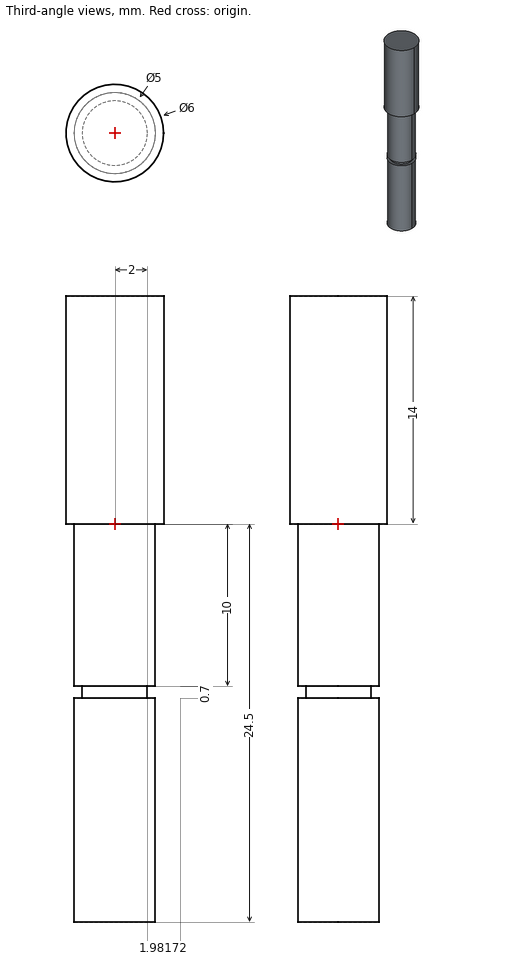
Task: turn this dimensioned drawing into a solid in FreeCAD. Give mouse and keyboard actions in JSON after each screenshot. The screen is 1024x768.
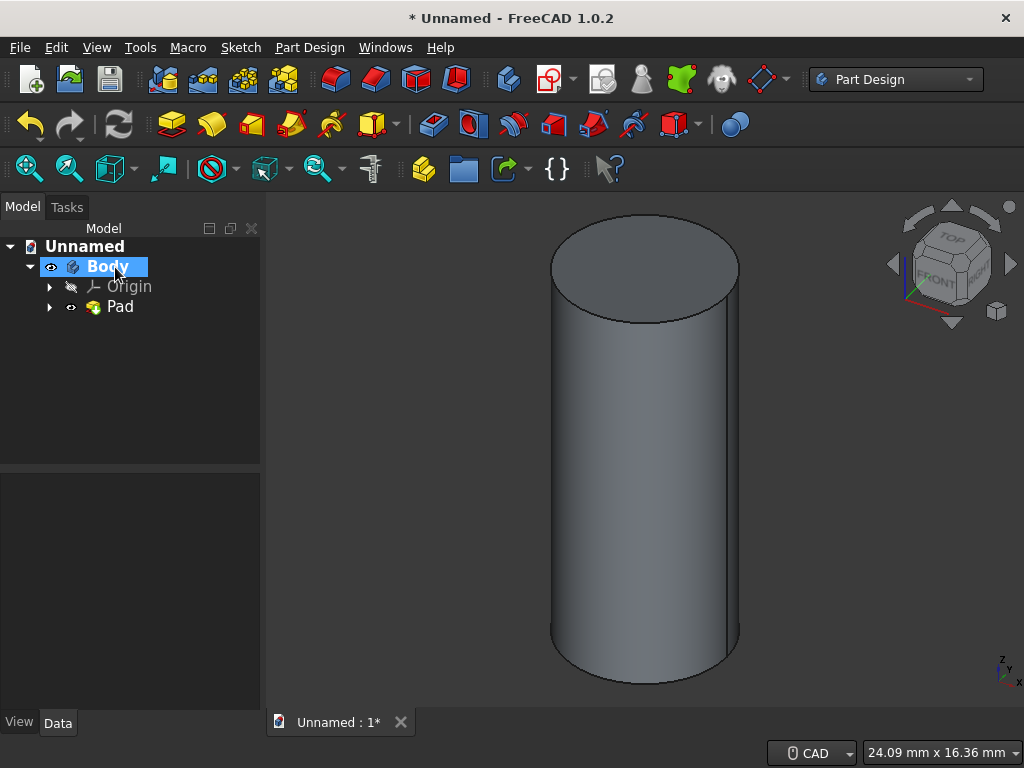
{"action": "left_click", "coordinate": [550, 80]}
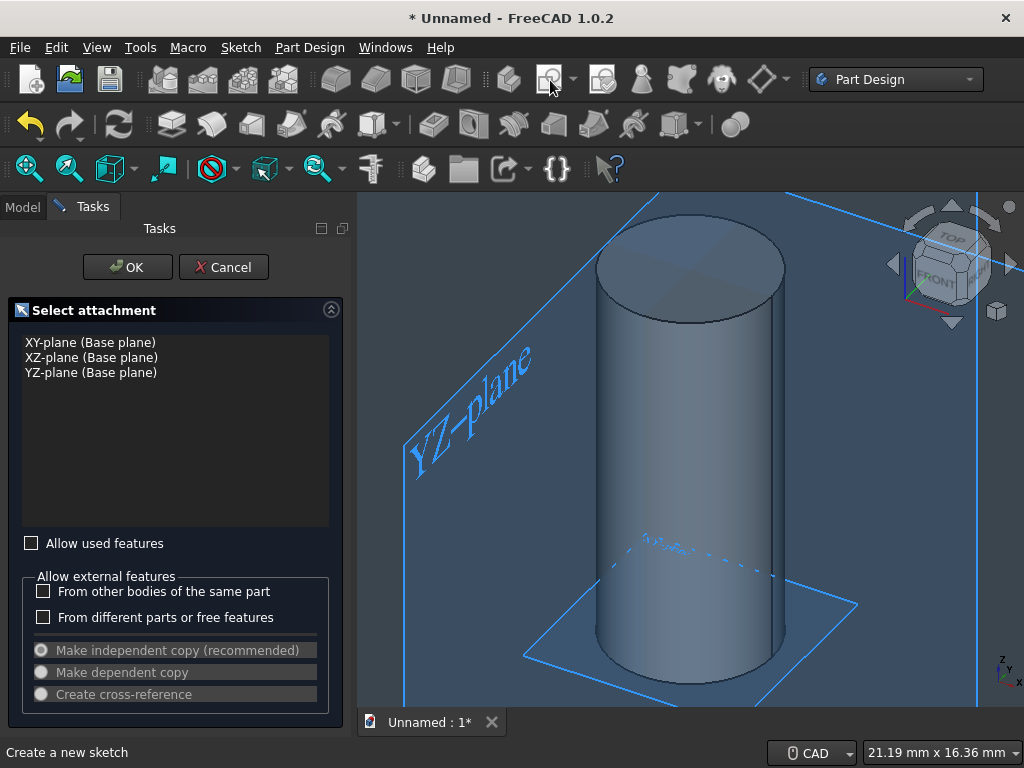
{"action": "left_click", "coordinate": [82, 342]}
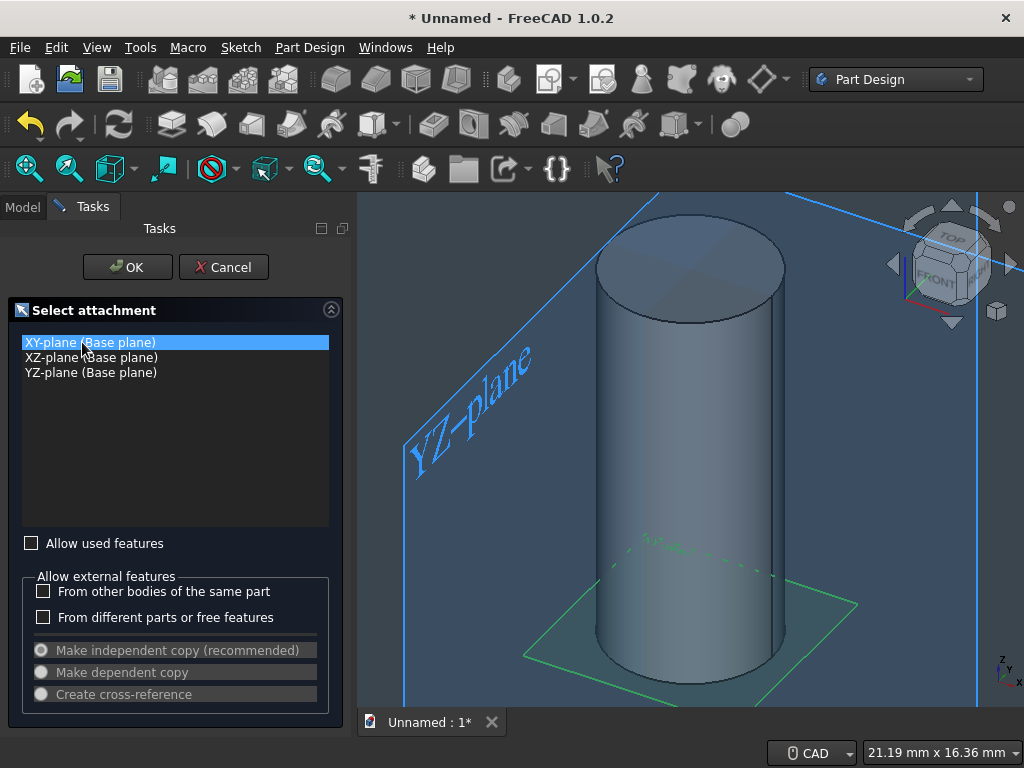
{"action": "left_click", "coordinate": [128, 267]}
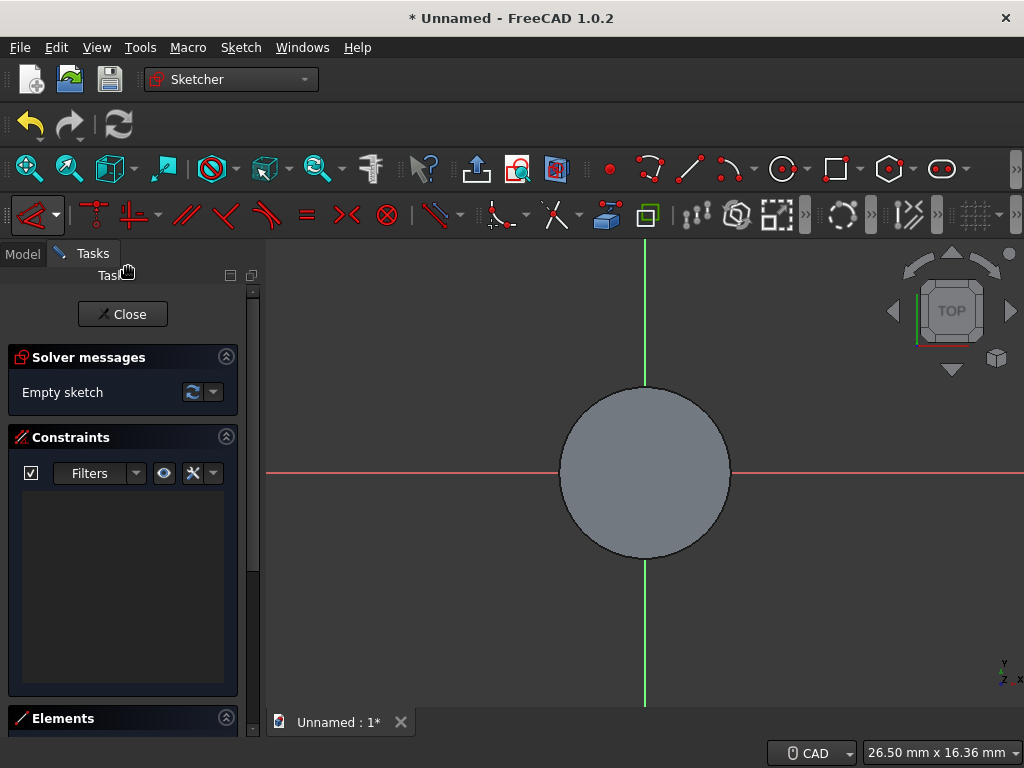
{"action": "left_click", "coordinate": [558, 170]}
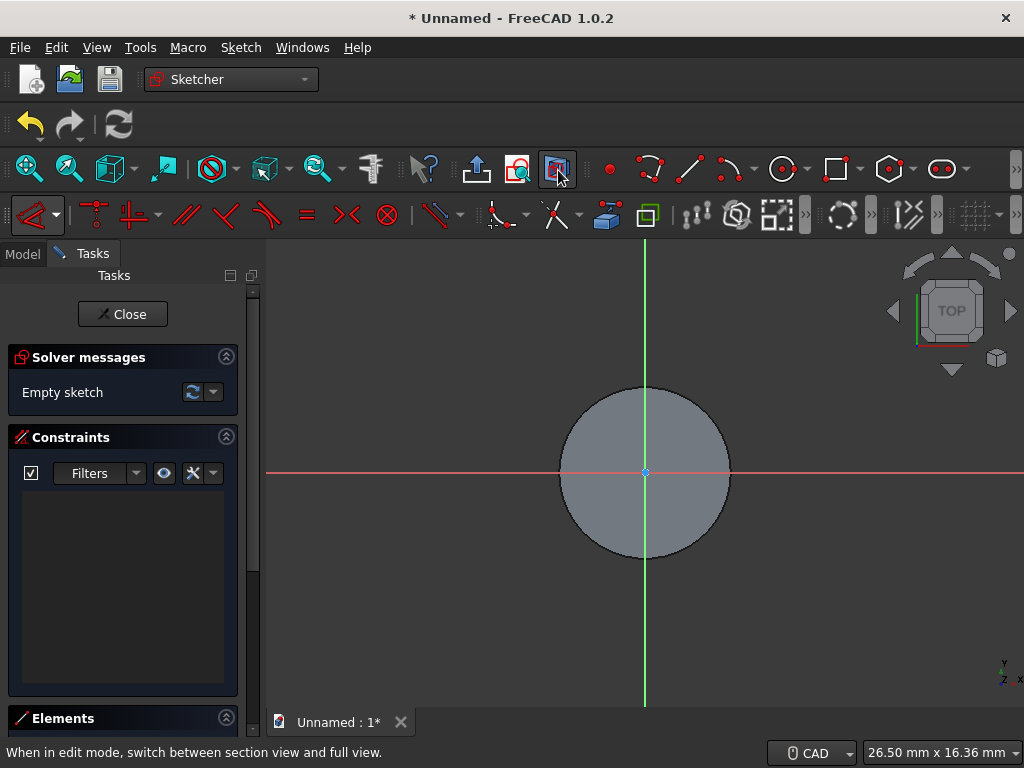
{"action": "scroll", "coordinate": [701, 473], "scroll_direction": "up", "scroll_amount": 4}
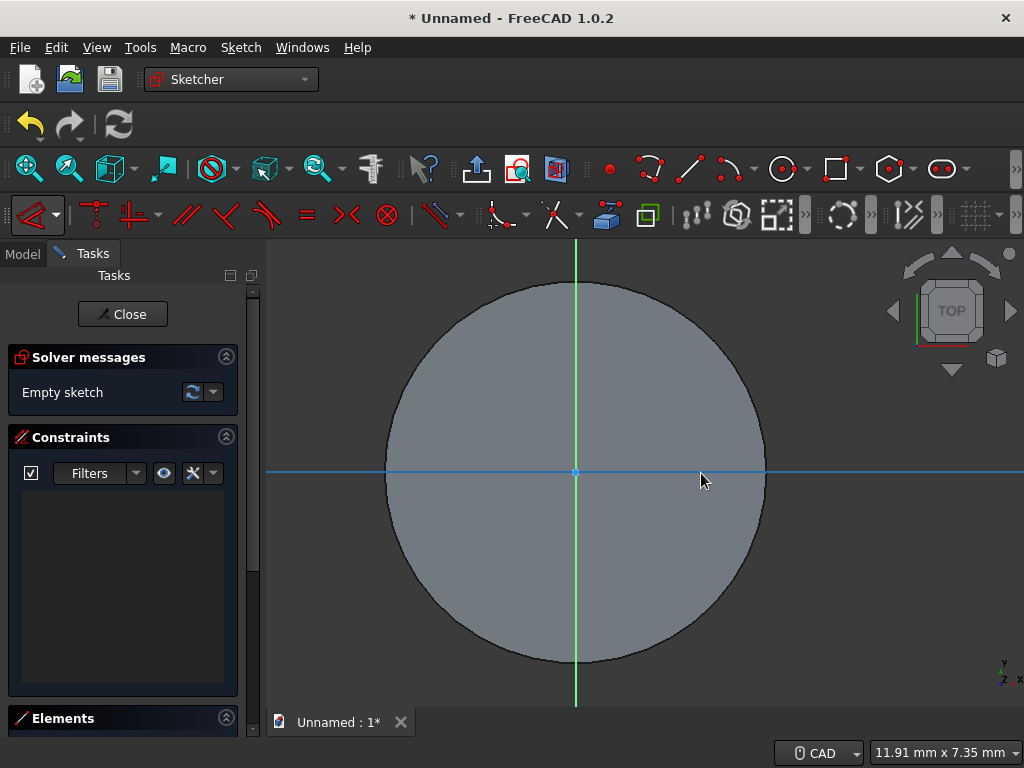
{"action": "left_click", "coordinate": [784, 170]}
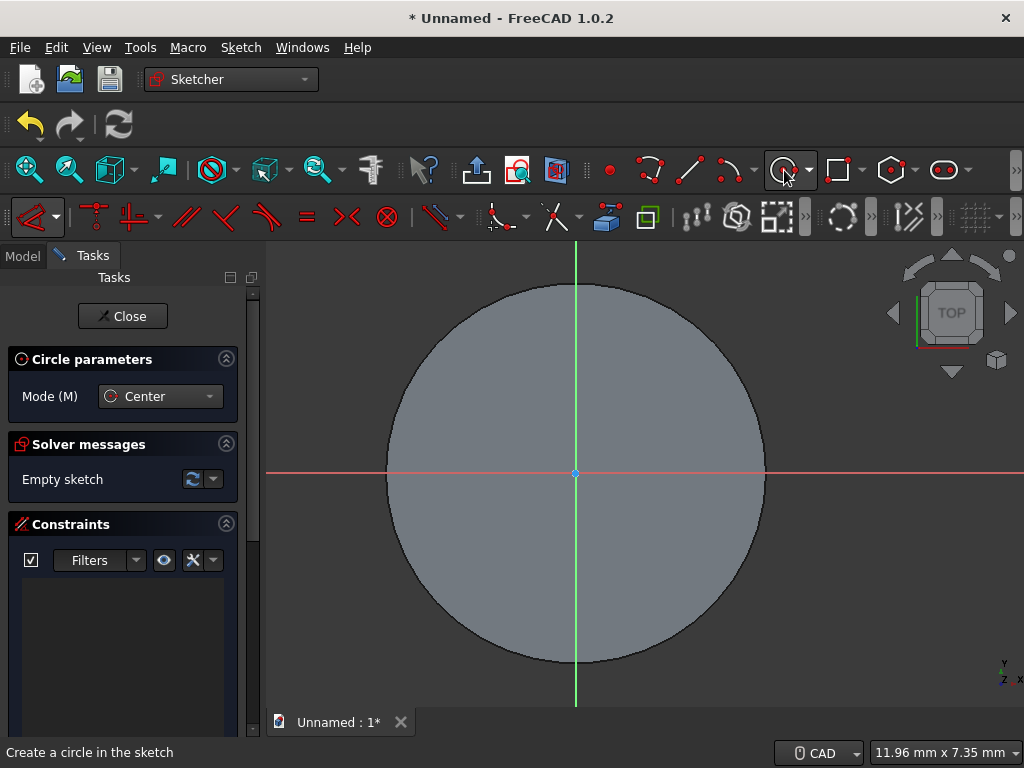
{"action": "left_click", "coordinate": [576, 473]}
{"action": "mouse_move", "coordinate": [688, 361]}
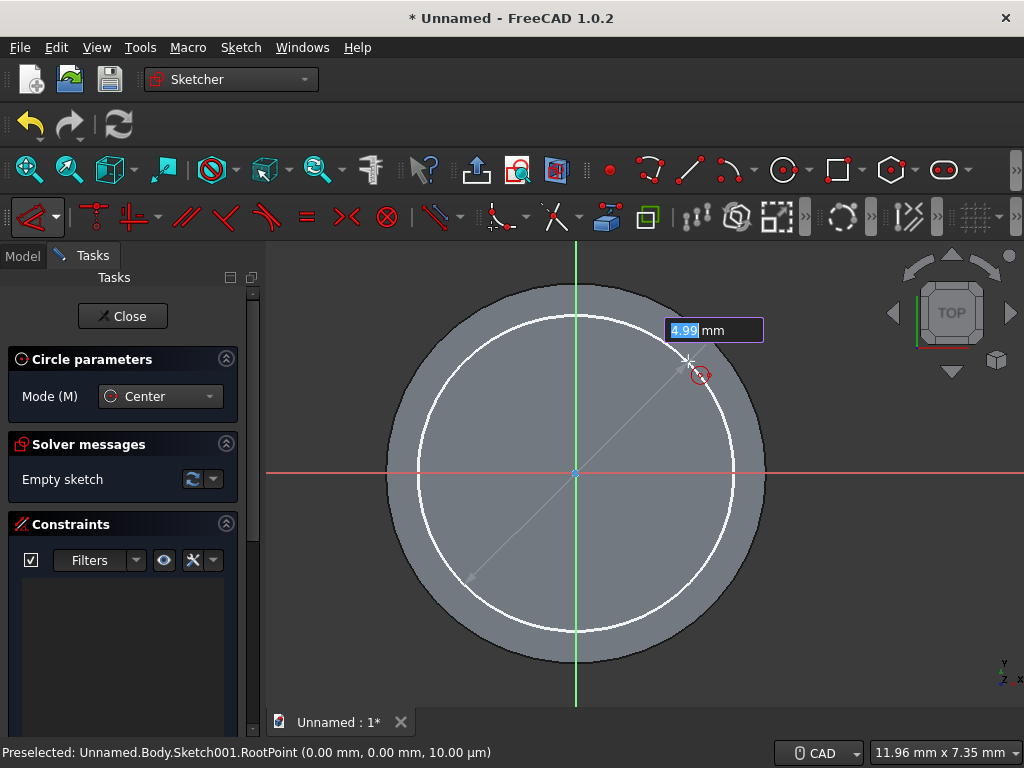
{"action": "type", "text": "5"}
{"action": "key", "text": "Return"}
{"action": "key", "text": "Escape"}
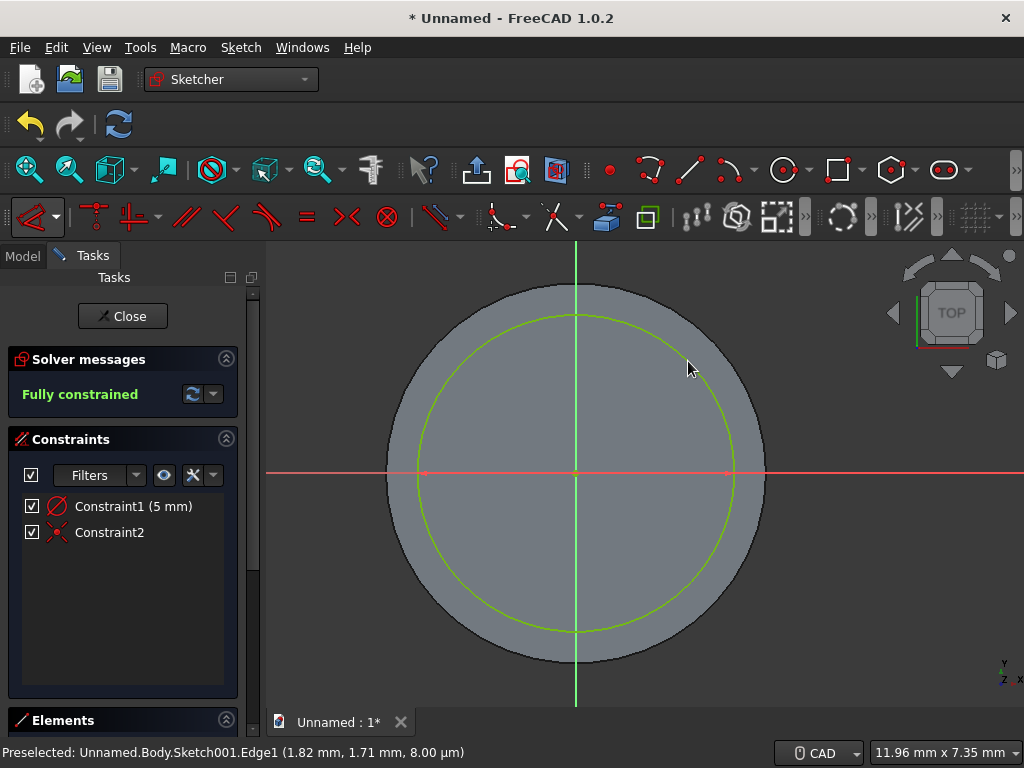
{"action": "left_click", "coordinate": [123, 316]}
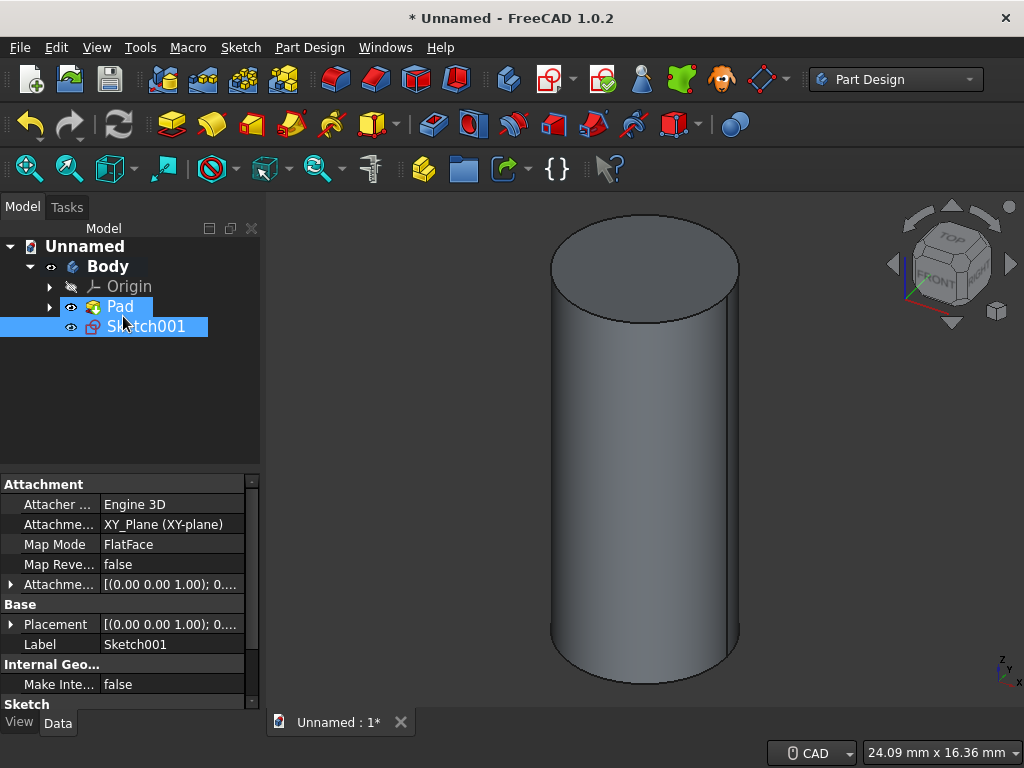
{"action": "left_click", "coordinate": [172, 124]}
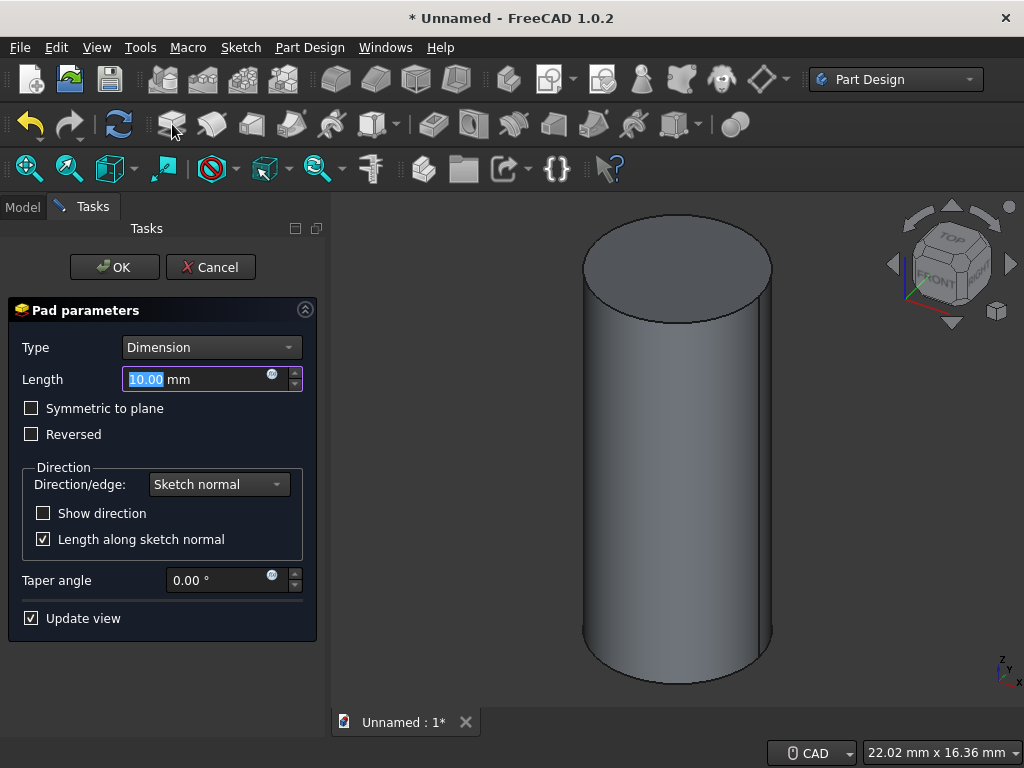
{"action": "type", "text": "24.5"}
{"action": "key", "text": "Tab"}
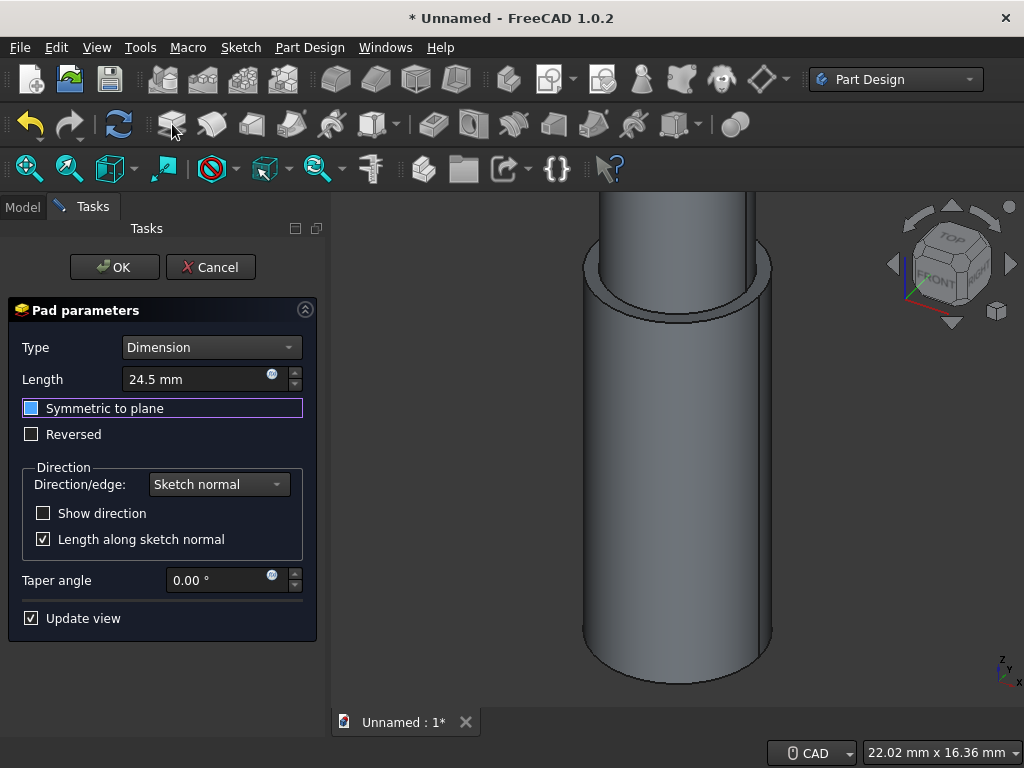
{"action": "left_click", "coordinate": [30, 434]}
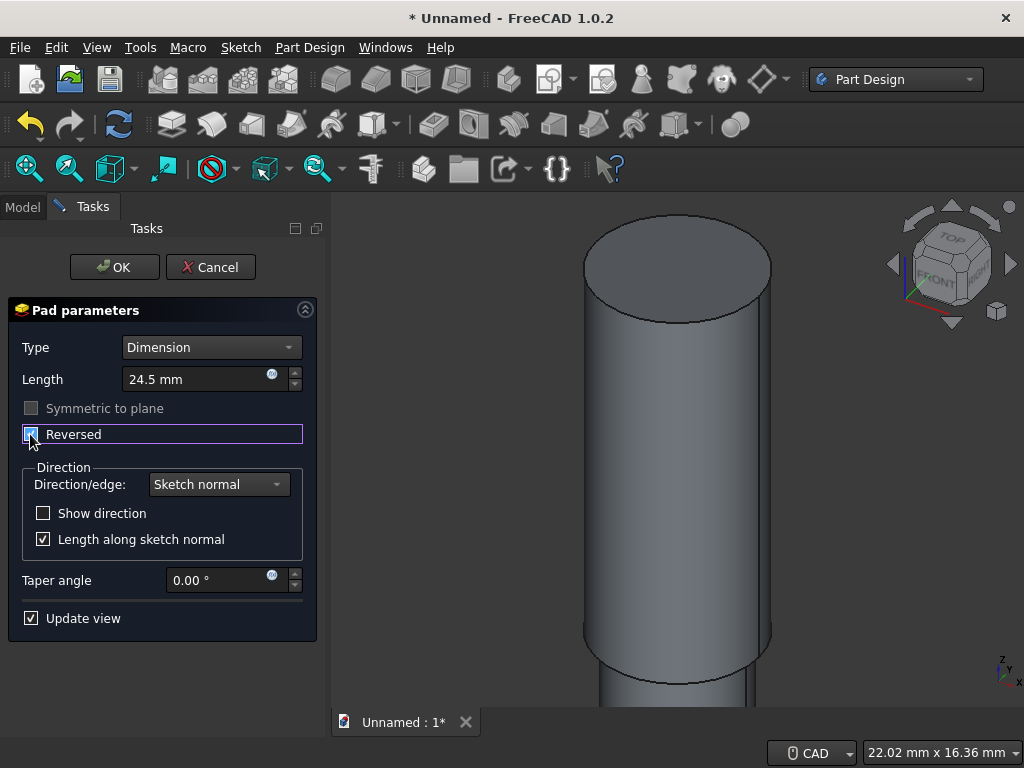
{"action": "left_click", "coordinate": [115, 267]}